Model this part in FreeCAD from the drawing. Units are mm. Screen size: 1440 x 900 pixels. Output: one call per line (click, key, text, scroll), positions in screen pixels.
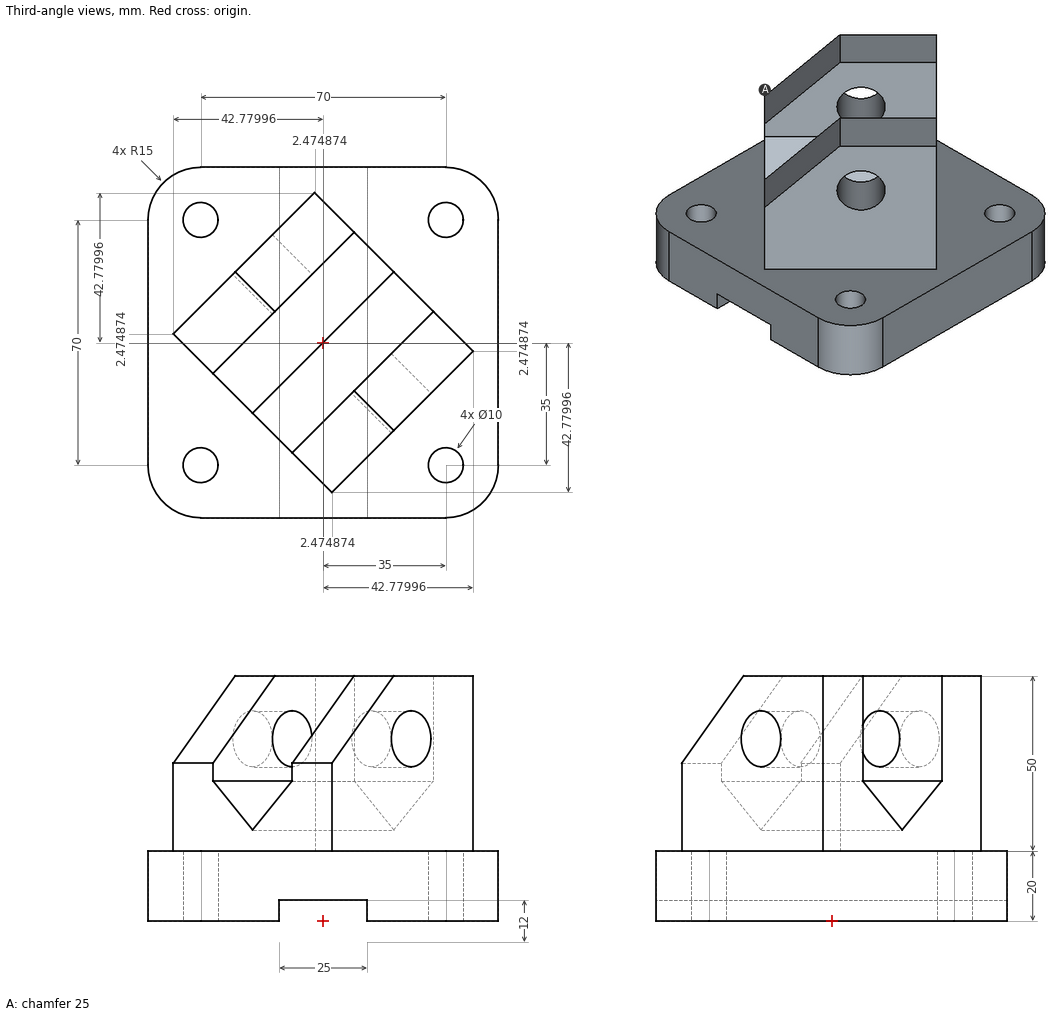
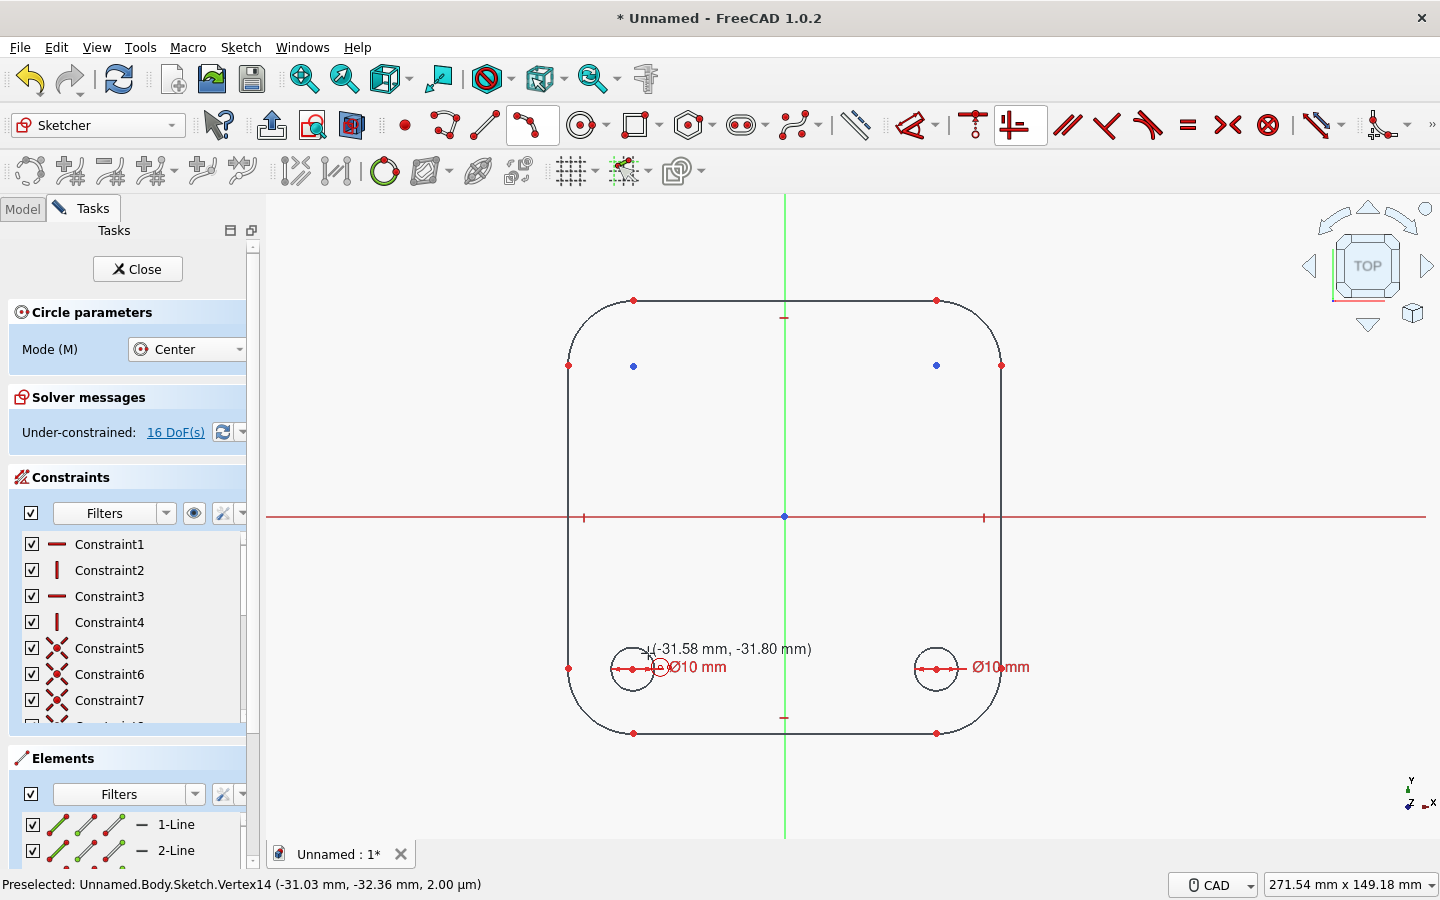
click(936, 365)
move(951, 350)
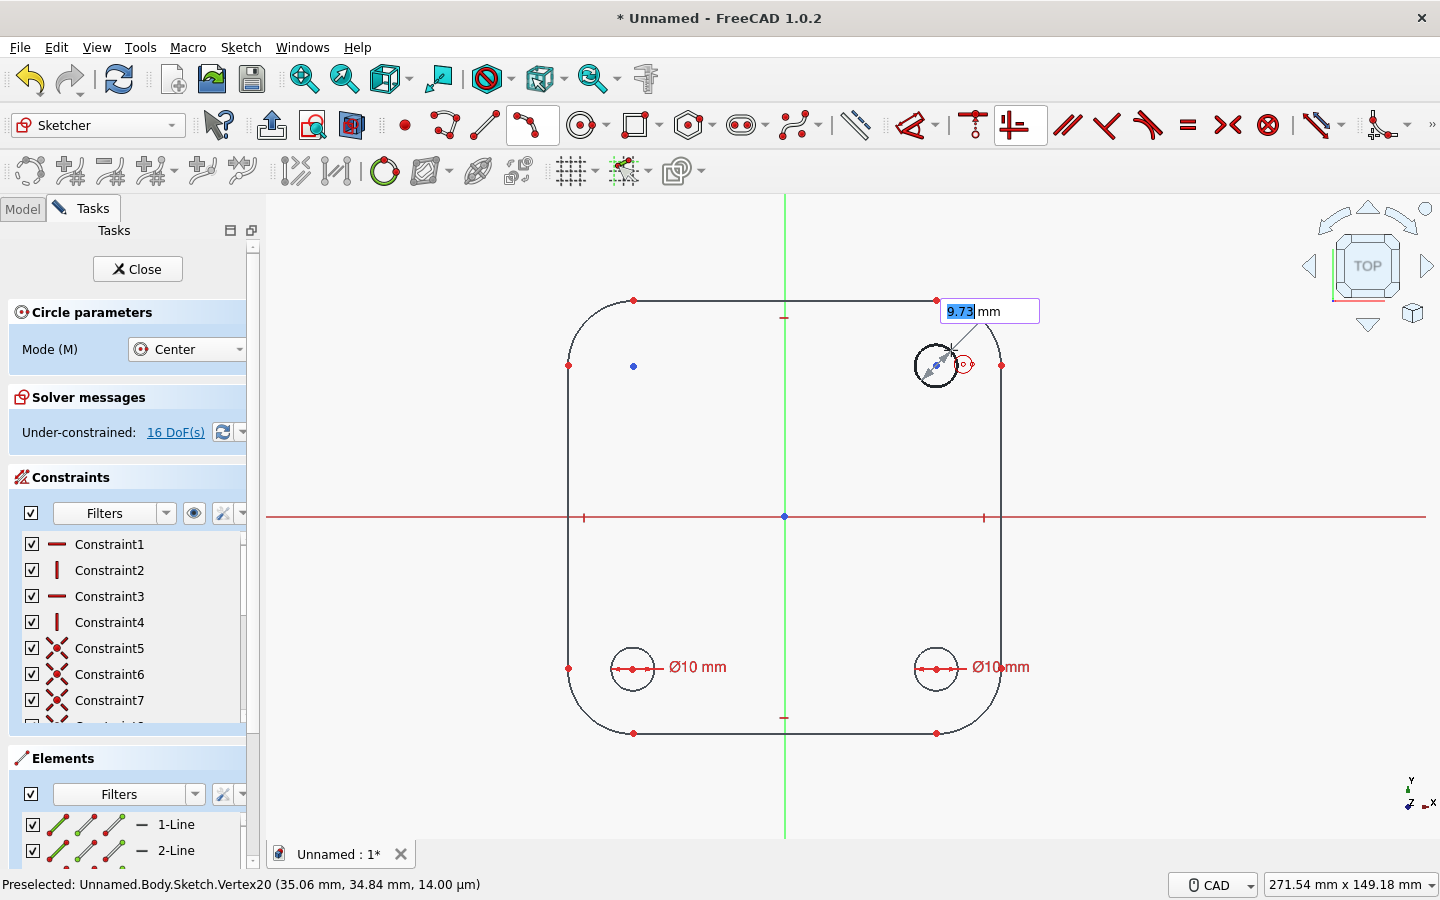
text(10)
key(Return)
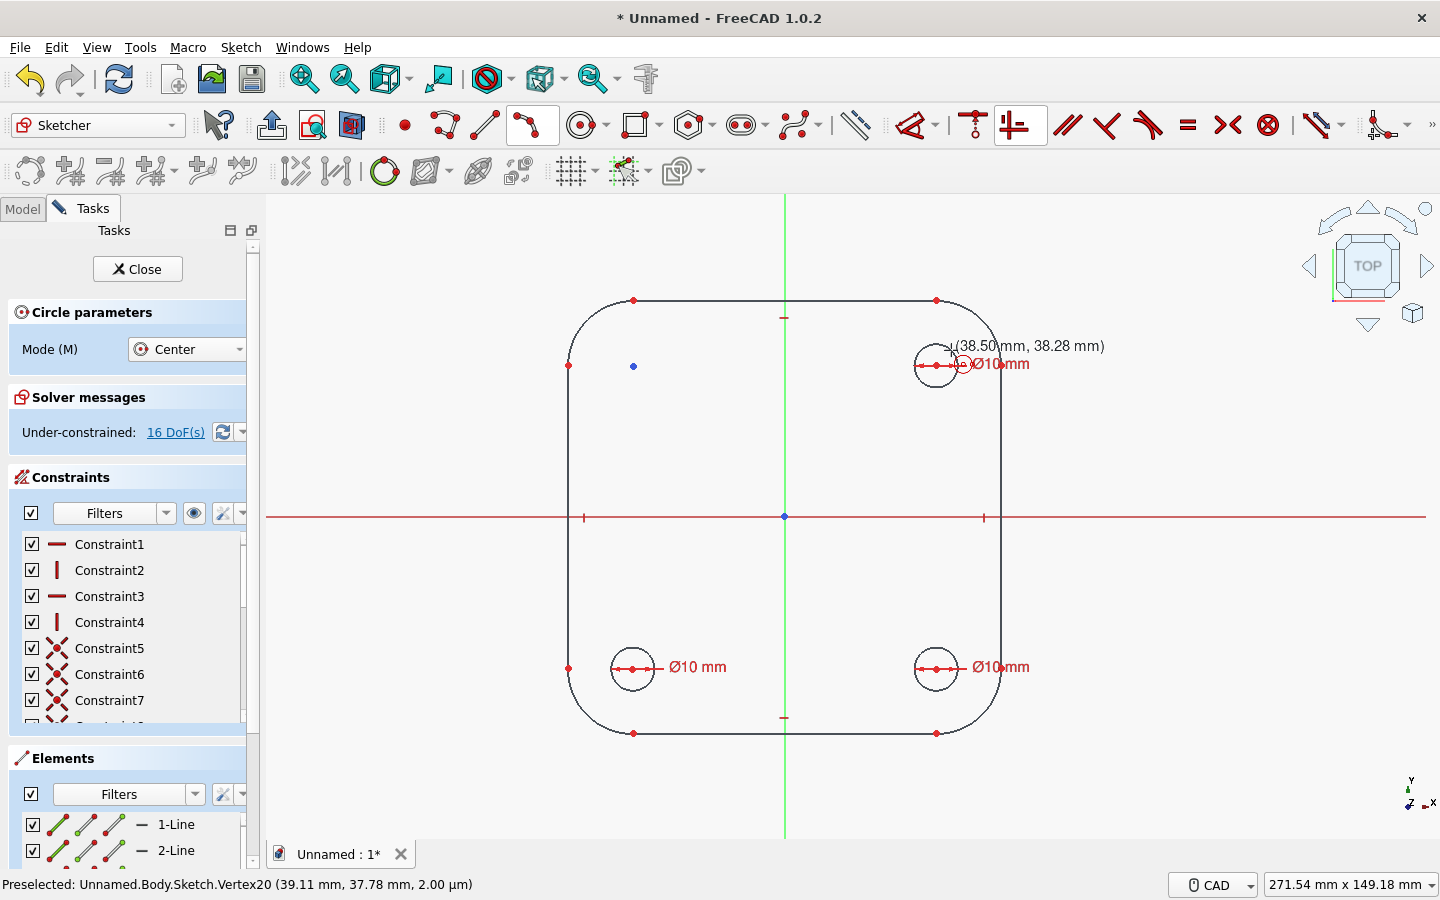
click(633, 365)
move(648, 350)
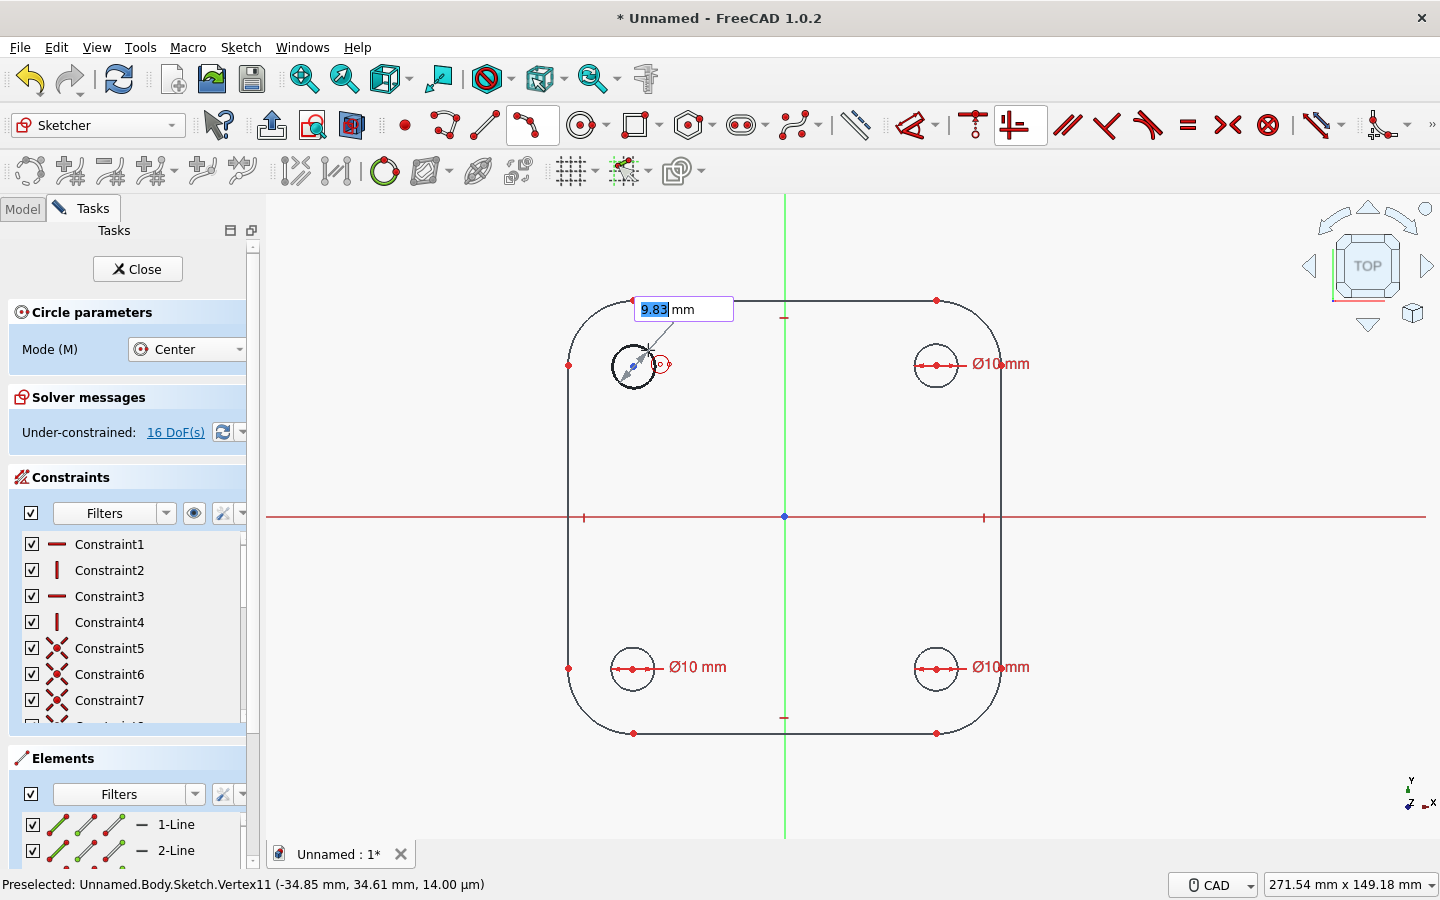
text(10)
key(Return)
key(Escape)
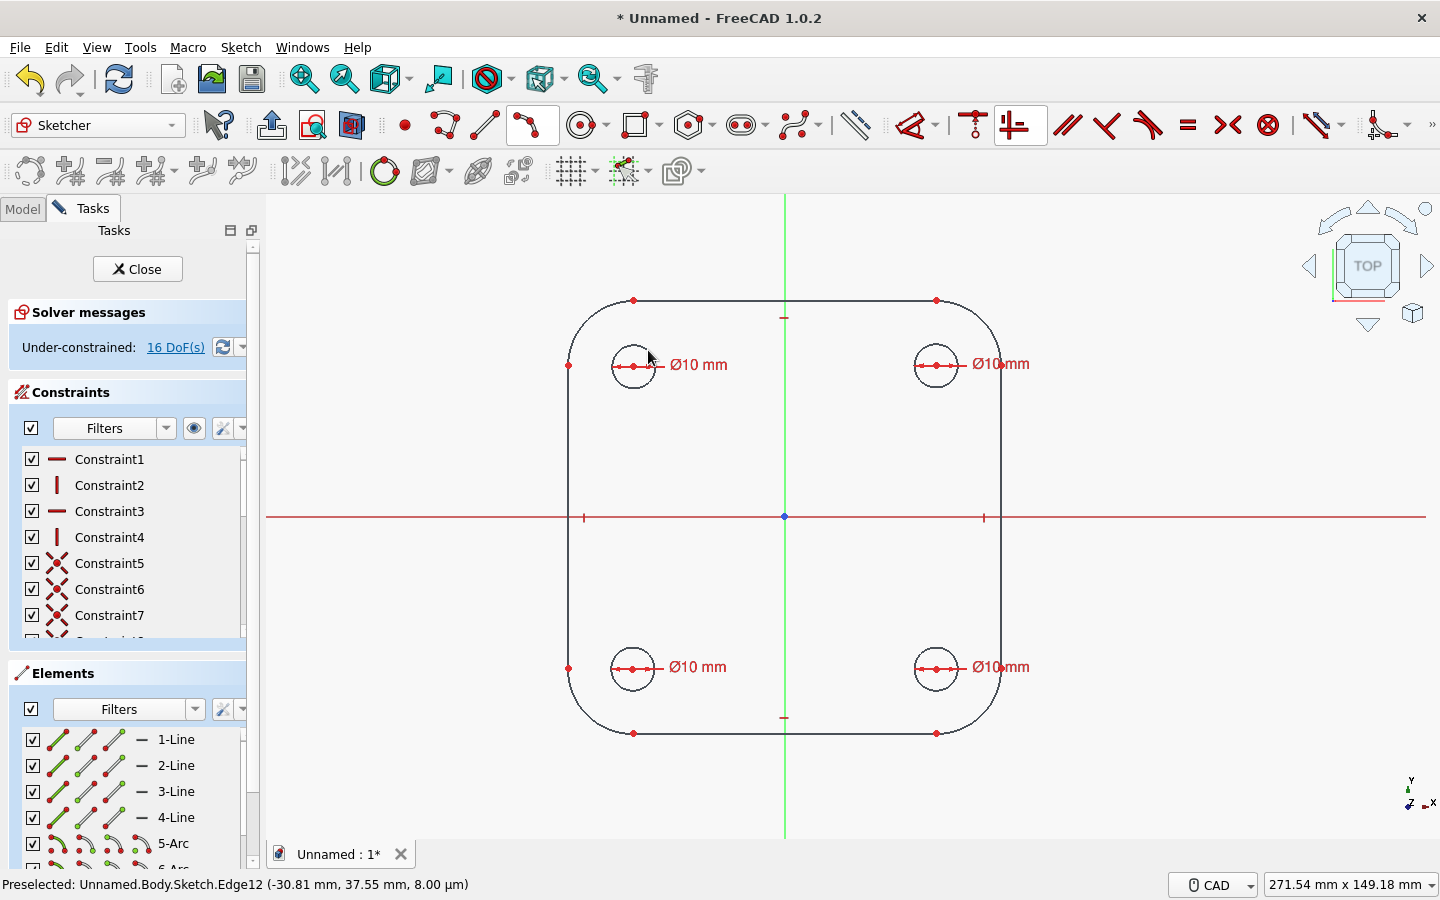
click(845, 301)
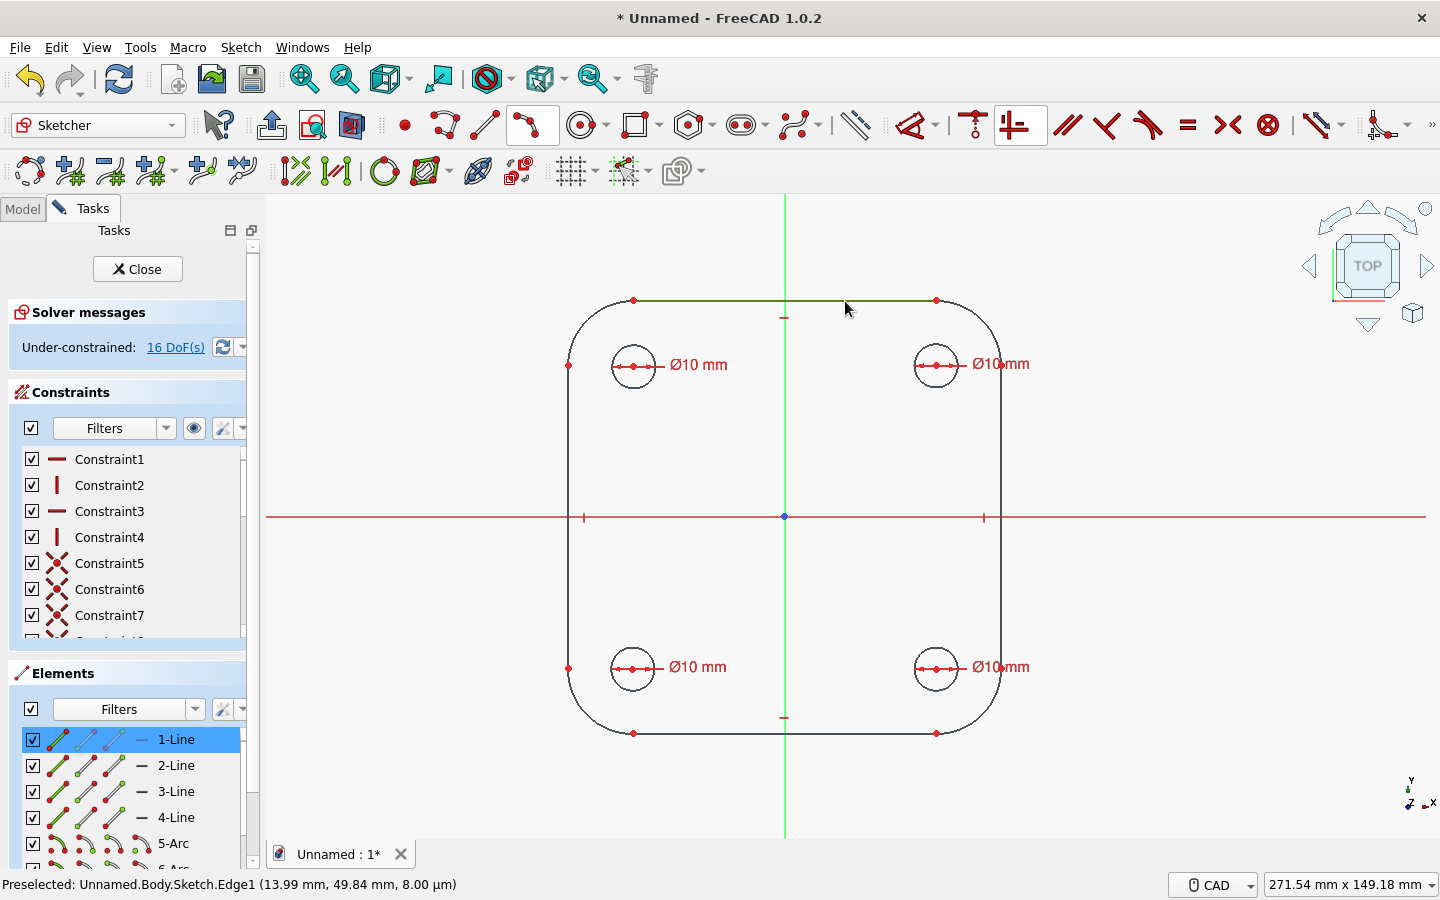
click(604, 308)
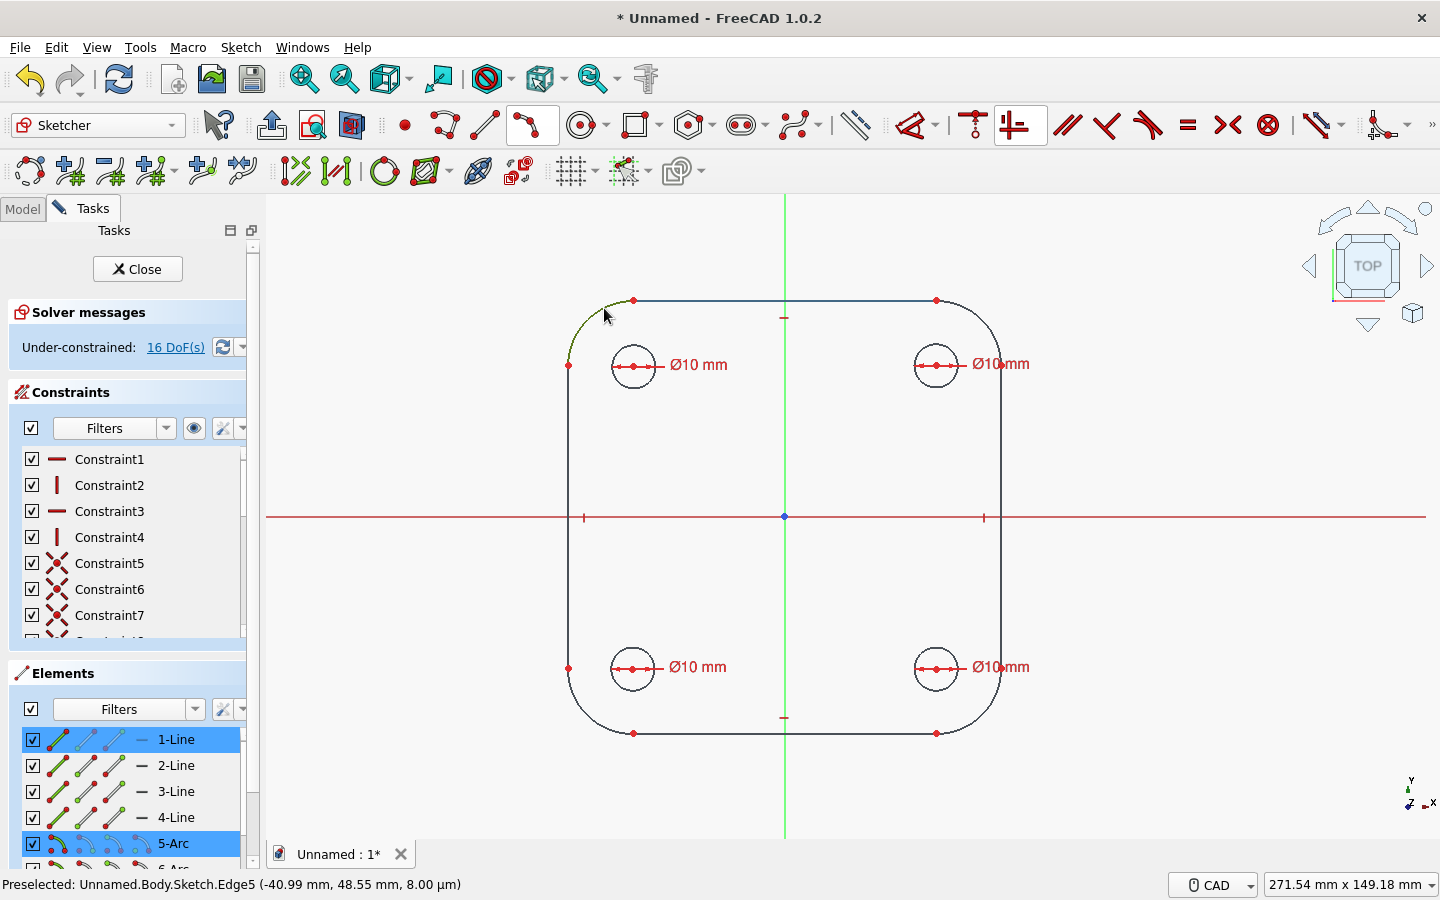
key(t)